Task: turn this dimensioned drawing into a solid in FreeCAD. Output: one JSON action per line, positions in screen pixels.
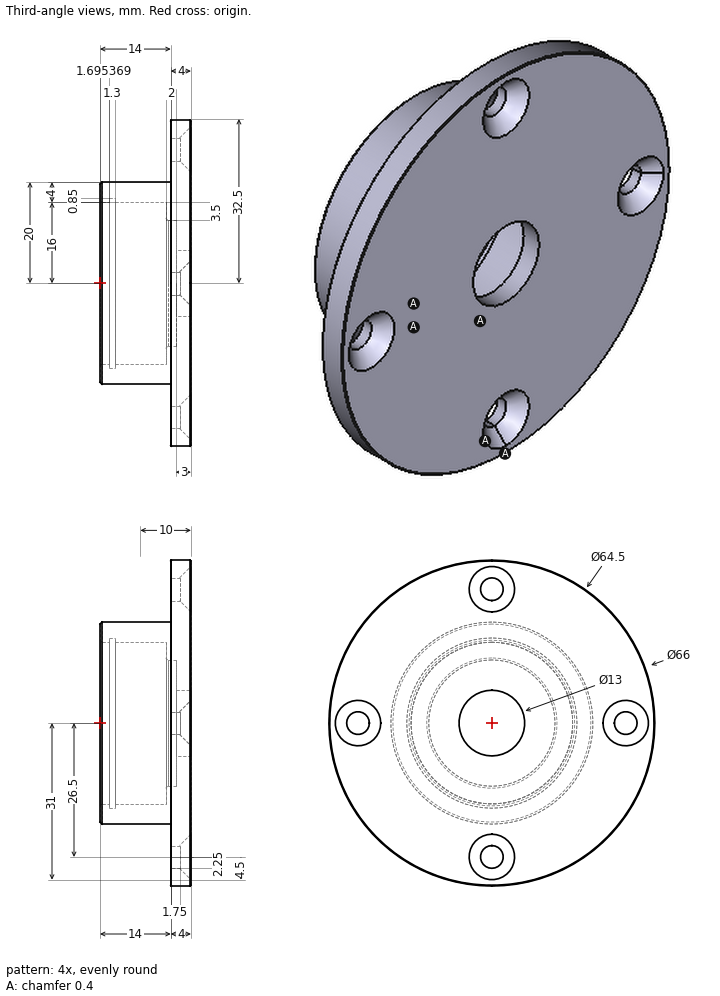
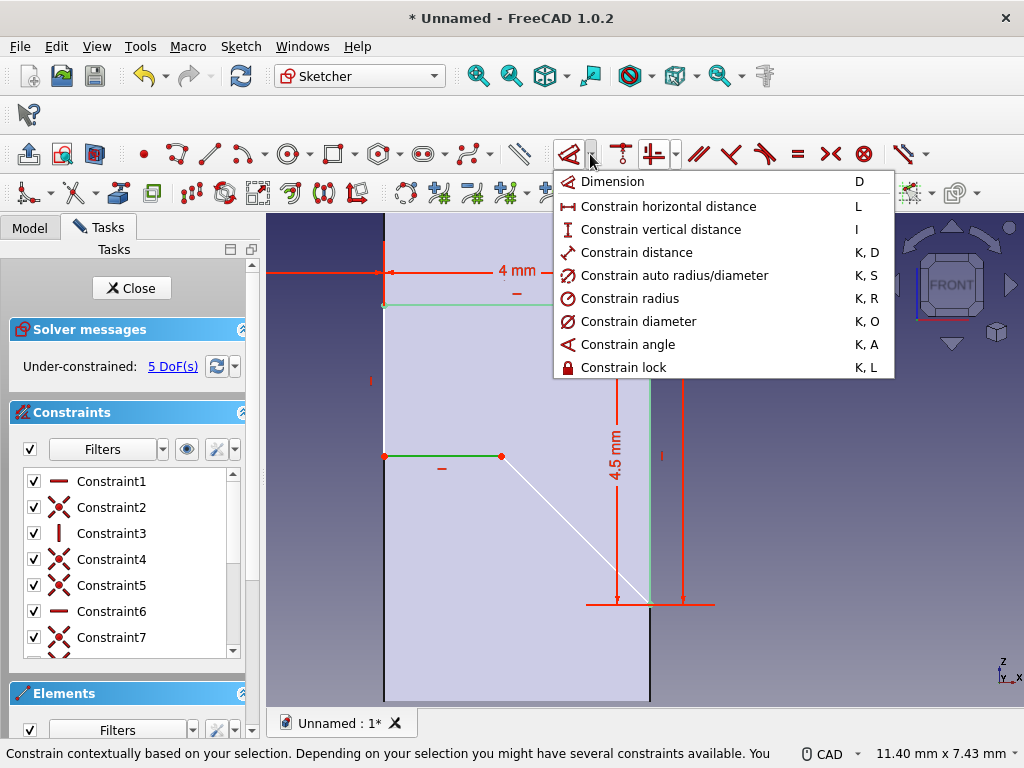
{"action": "left_click", "coordinate": [724, 206]}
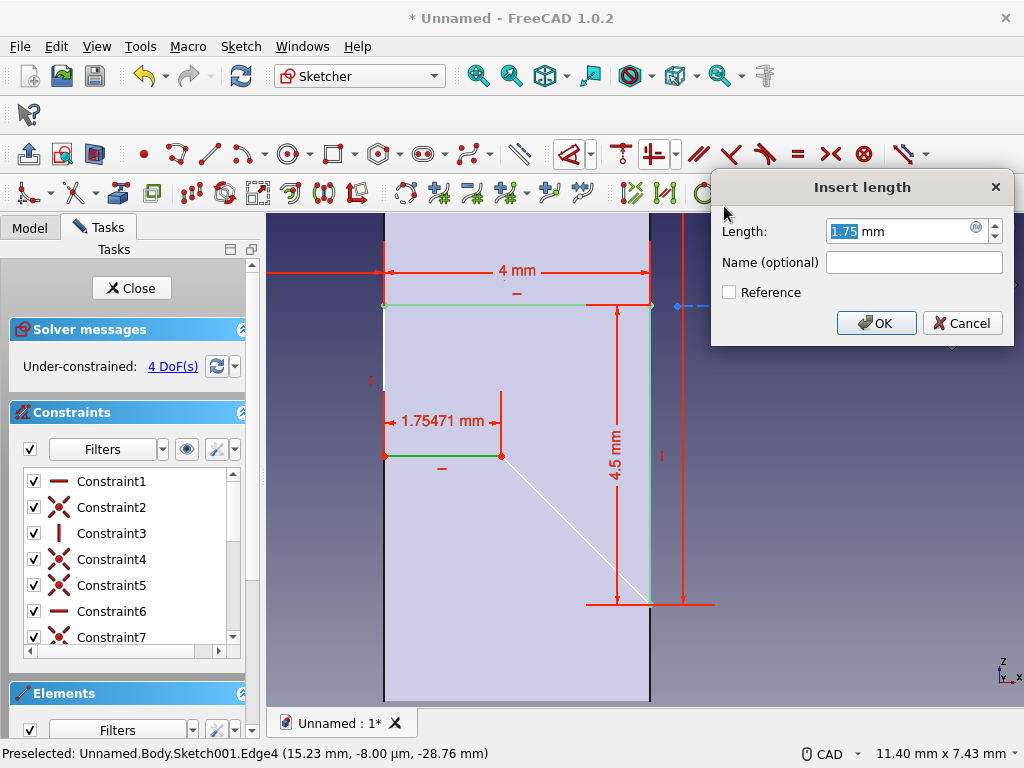
{"action": "type", "text": "1.75"}
{"action": "key", "text": "Return"}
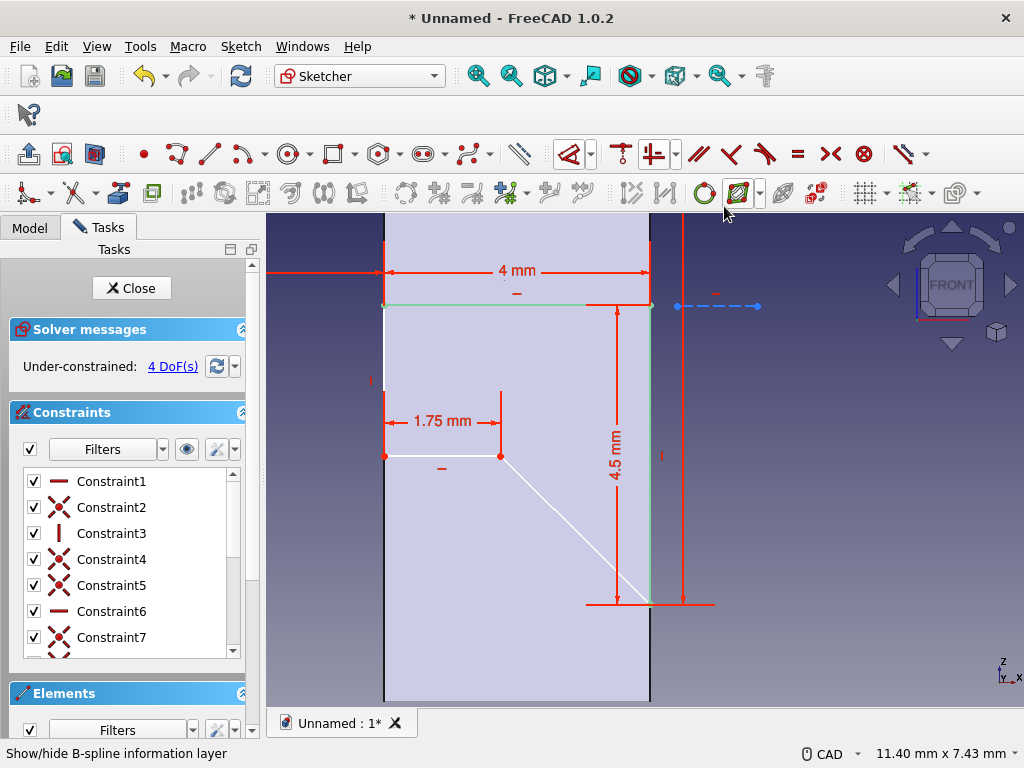
{"action": "left_click", "coordinate": [384, 411]}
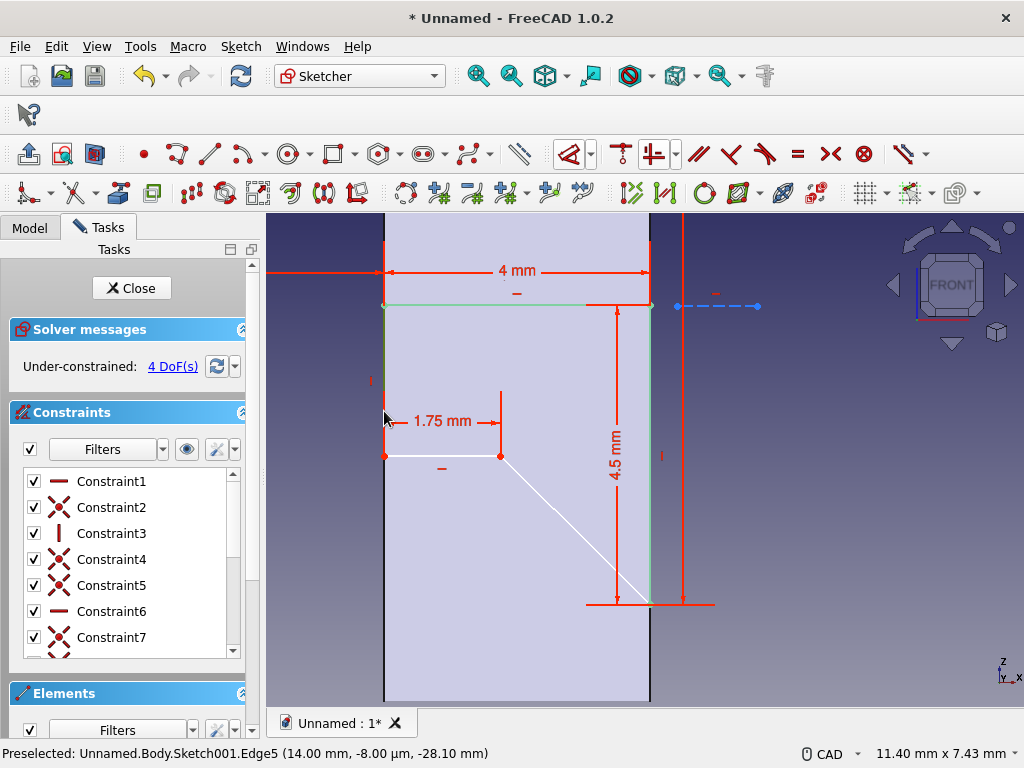
{"action": "left_click", "coordinate": [590, 154]}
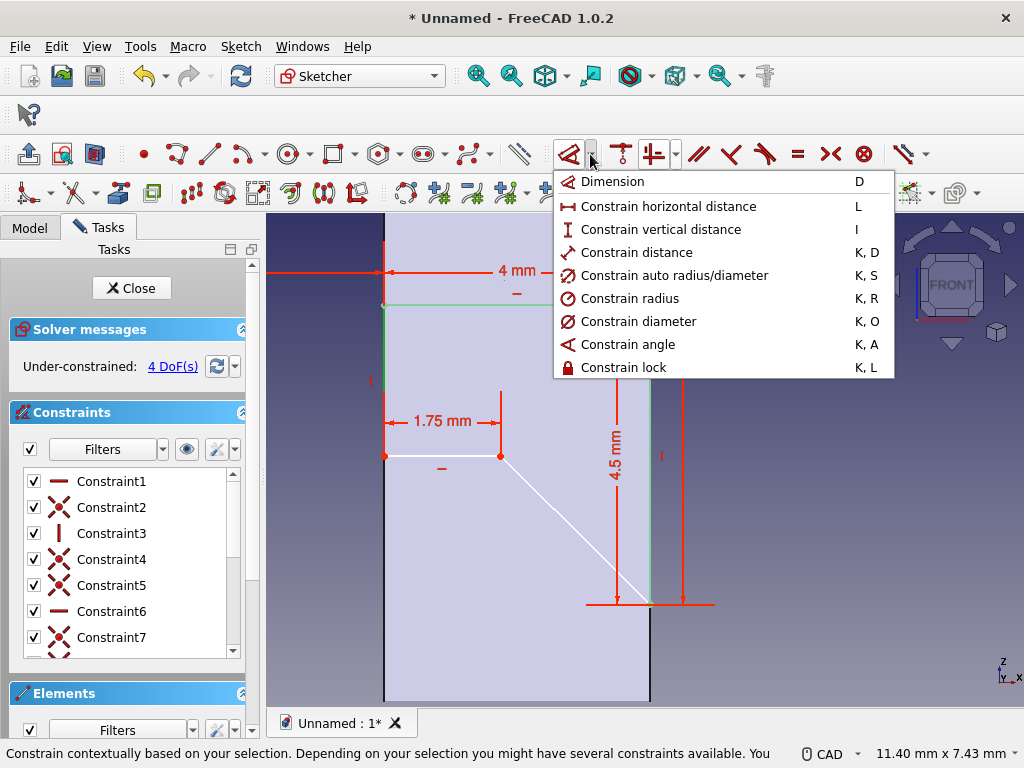
{"action": "left_click", "coordinate": [724, 230]}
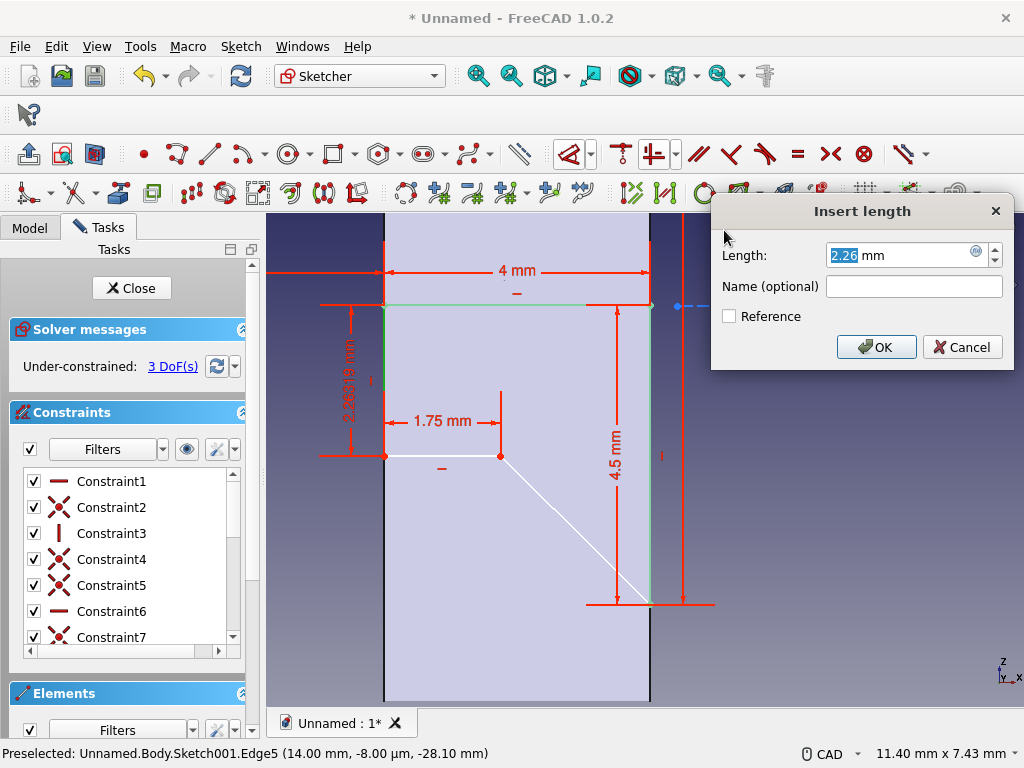
{"action": "type", "text": "2.25"}
{"action": "key", "text": "Return"}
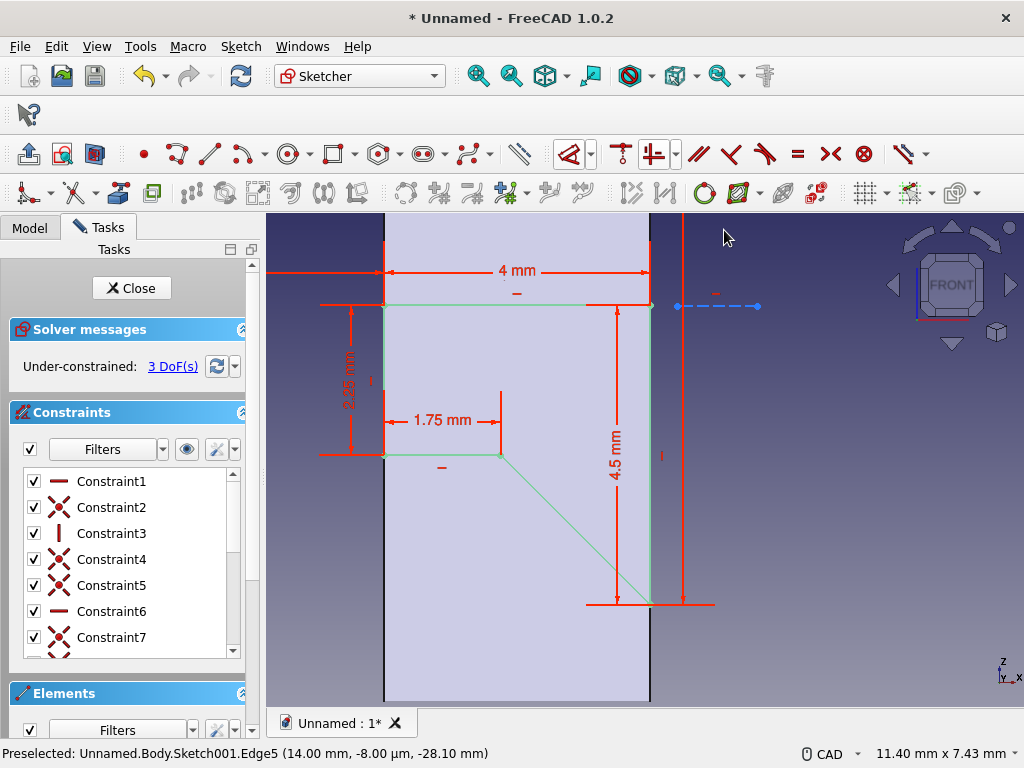
{"action": "left_click", "coordinate": [677, 306]}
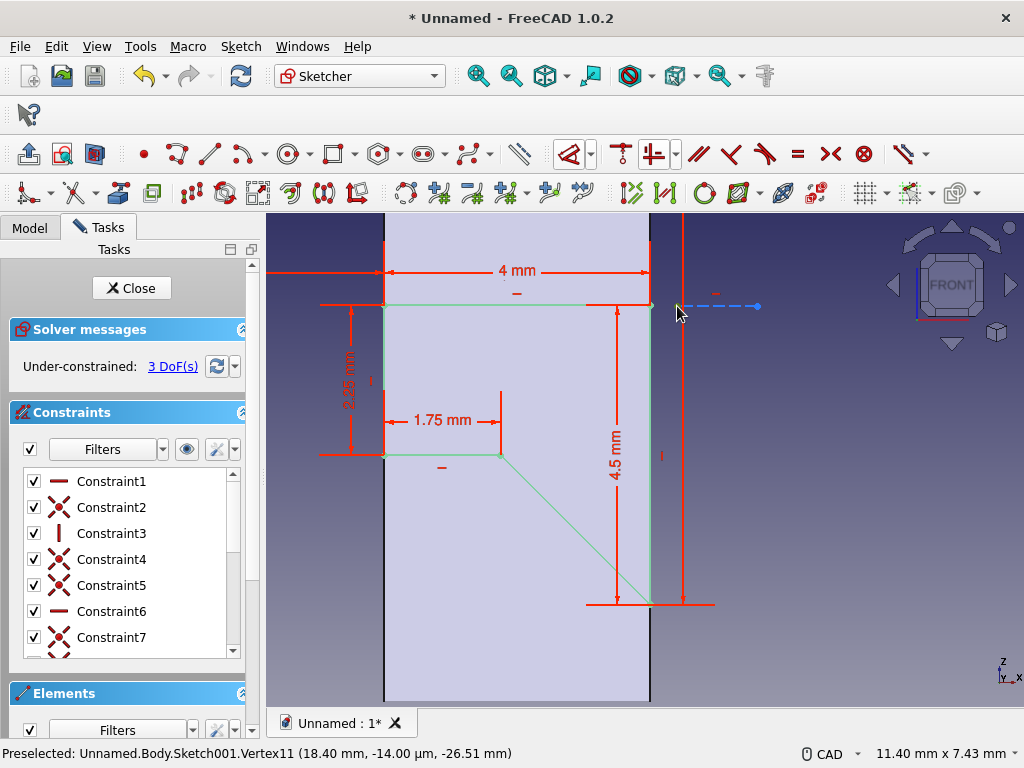
{"action": "left_click", "coordinate": [590, 154]}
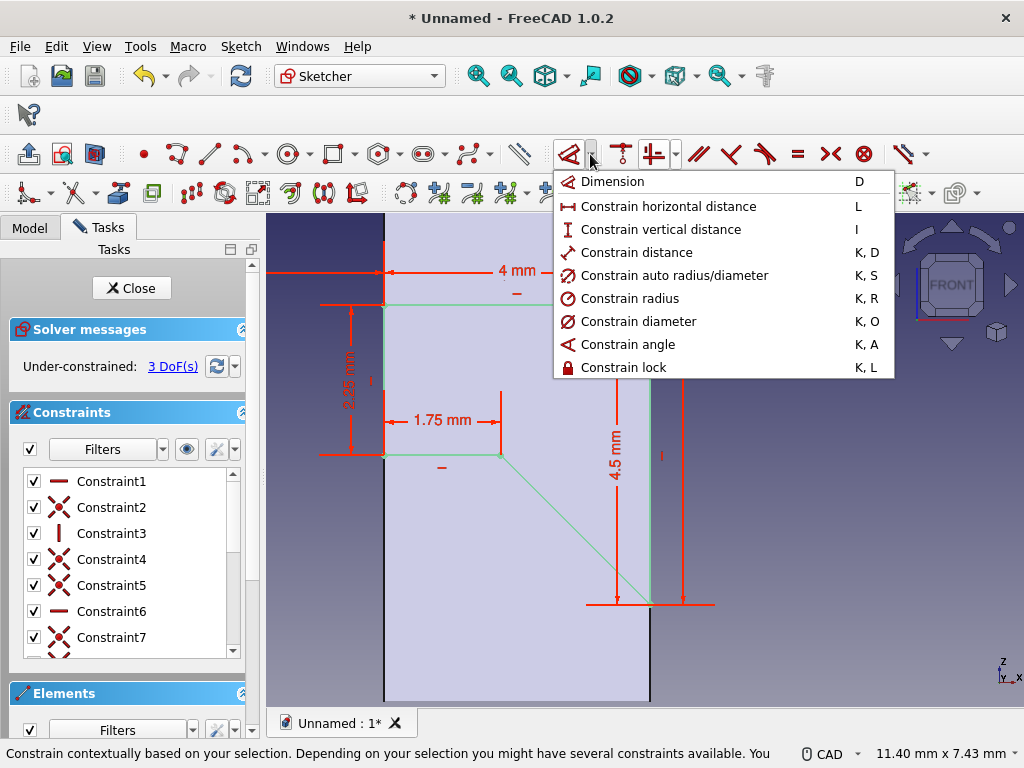
{"action": "left_click", "coordinate": [724, 230]}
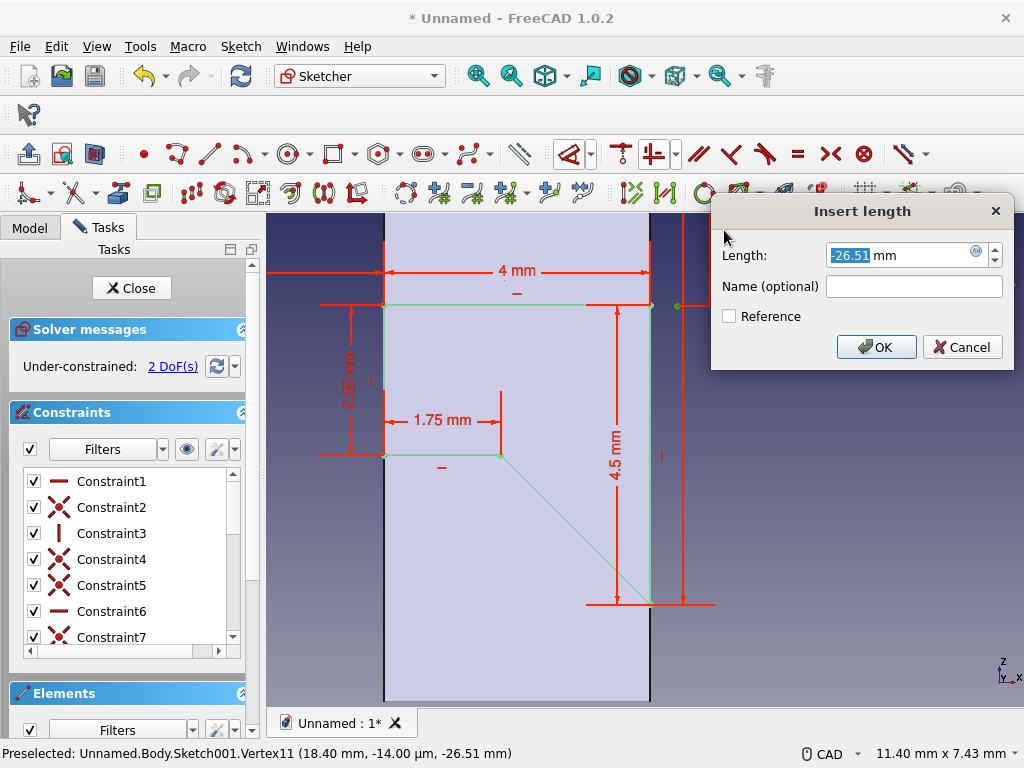
{"action": "type", "text": "-26.5"}
{"action": "key", "text": "Return"}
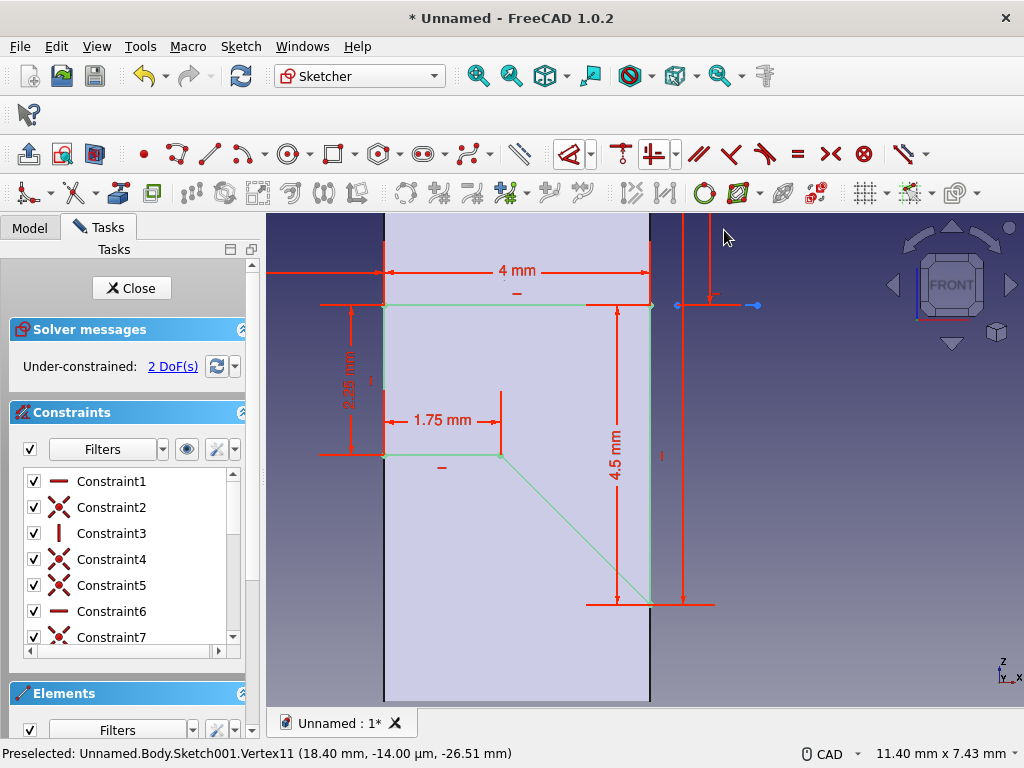
{"action": "left_click", "coordinate": [132, 288]}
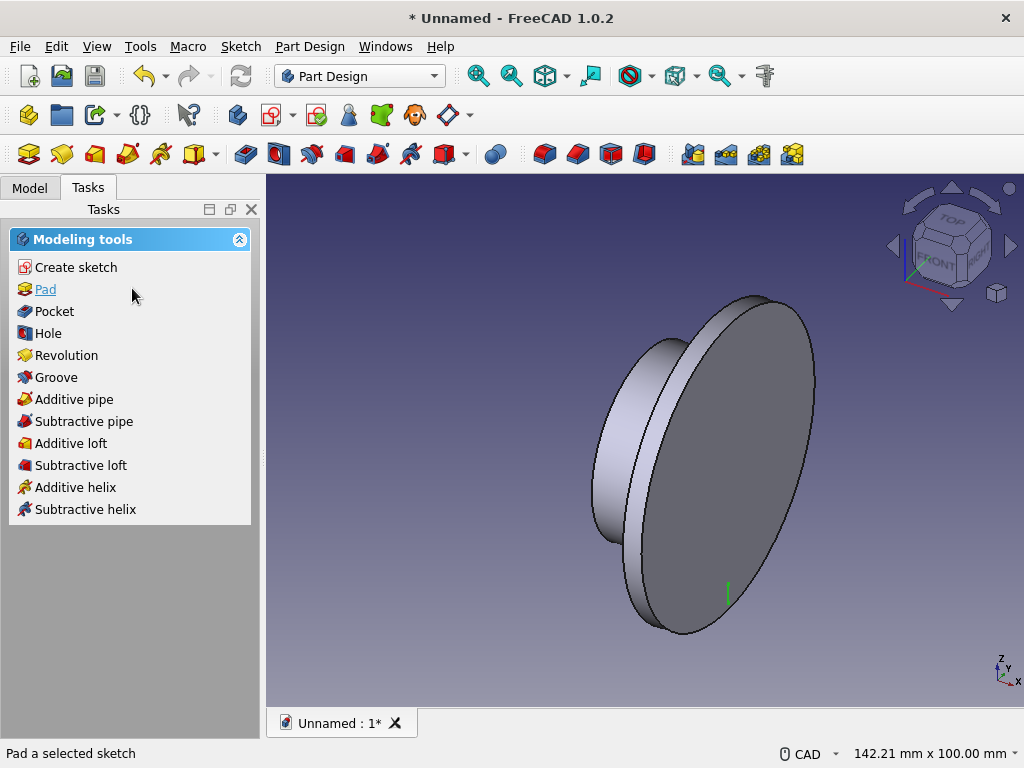
{"action": "left_click", "coordinate": [312, 154]}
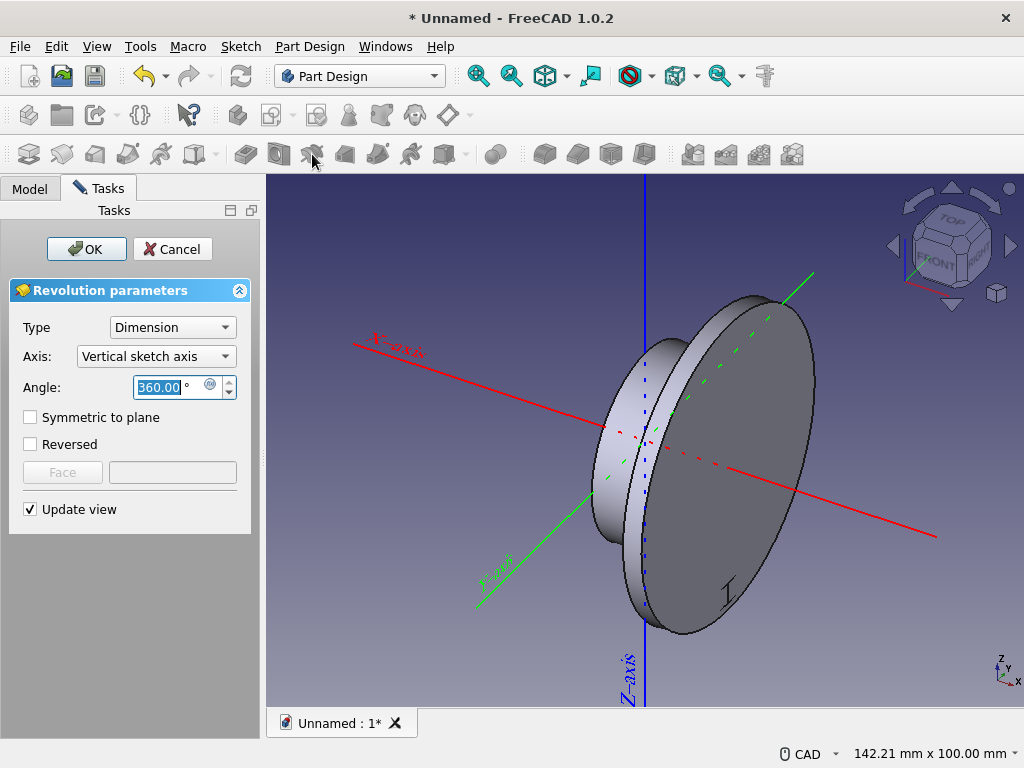
{"action": "left_click", "coordinate": [157, 356]}